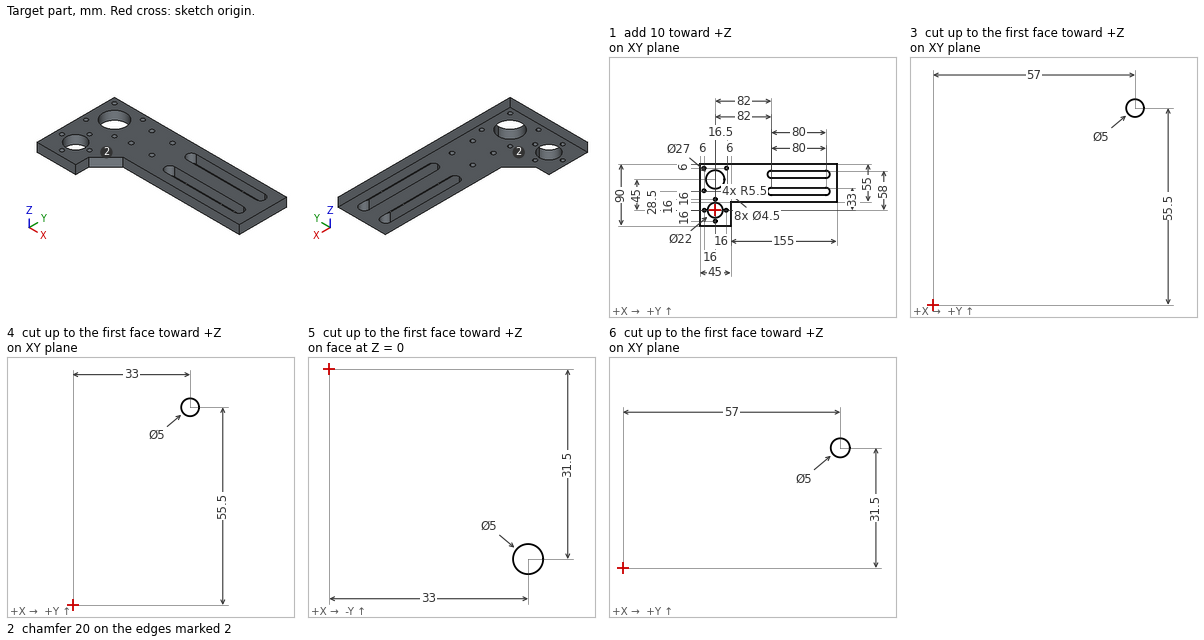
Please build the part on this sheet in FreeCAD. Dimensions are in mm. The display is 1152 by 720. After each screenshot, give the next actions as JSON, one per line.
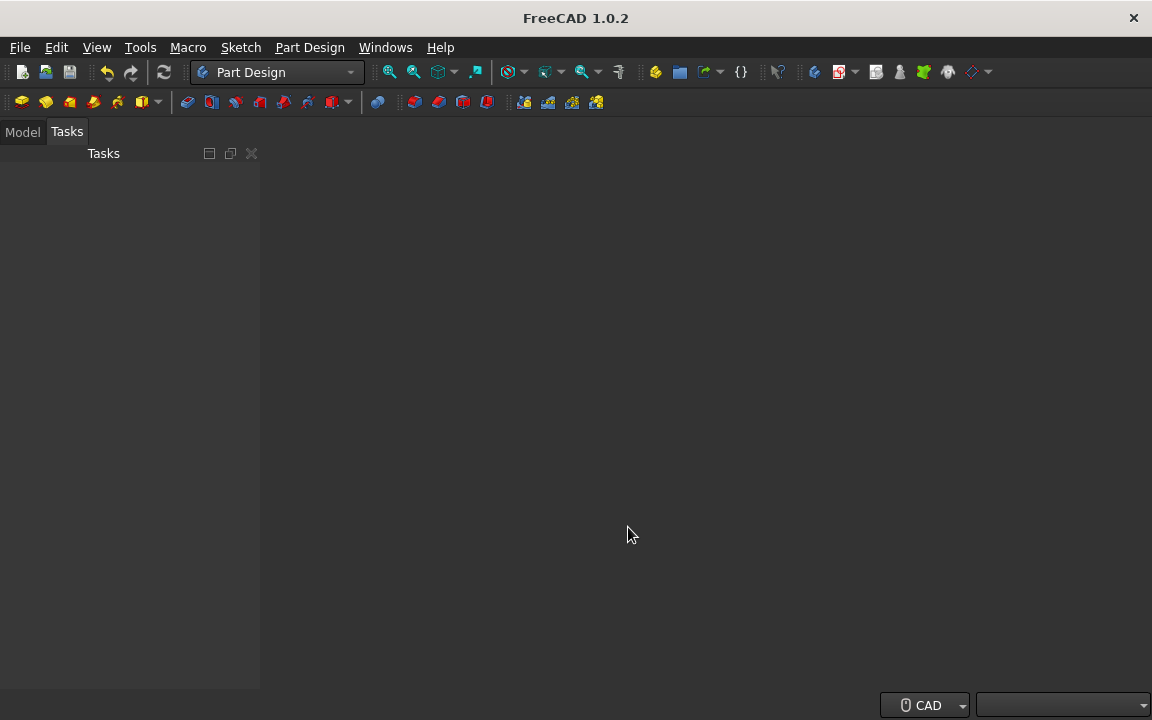
{"action": "key", "text": "ctrl+n"}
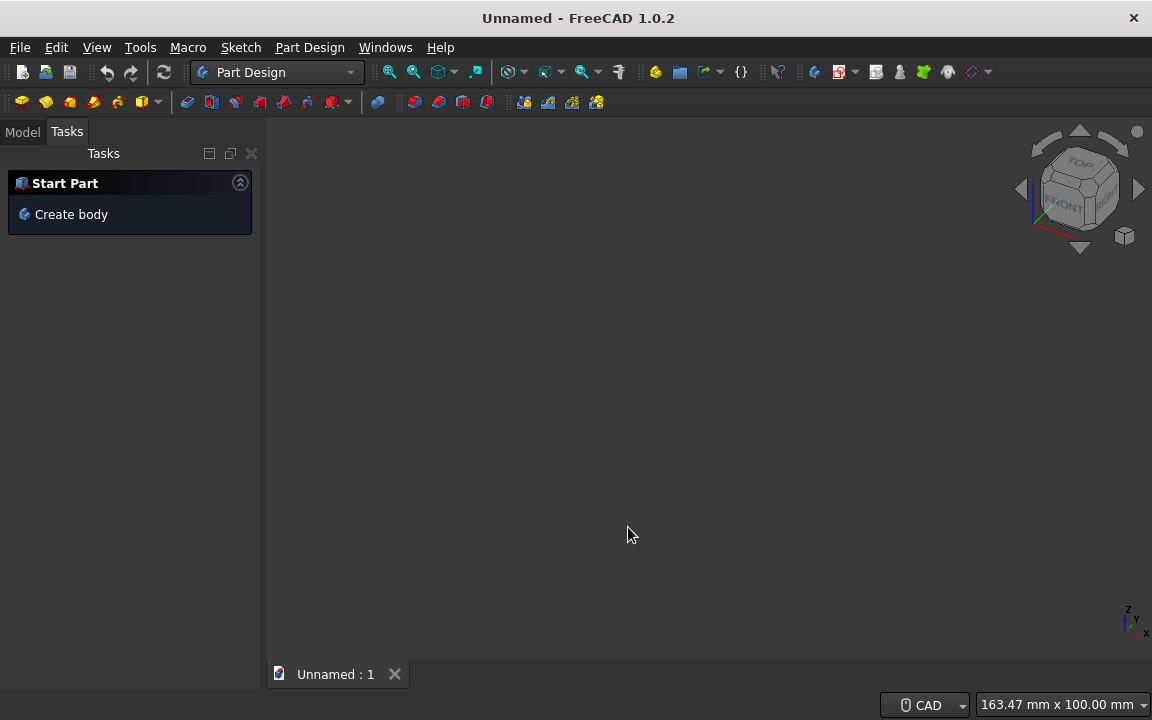
{"action": "left_click", "coordinate": [840, 72]}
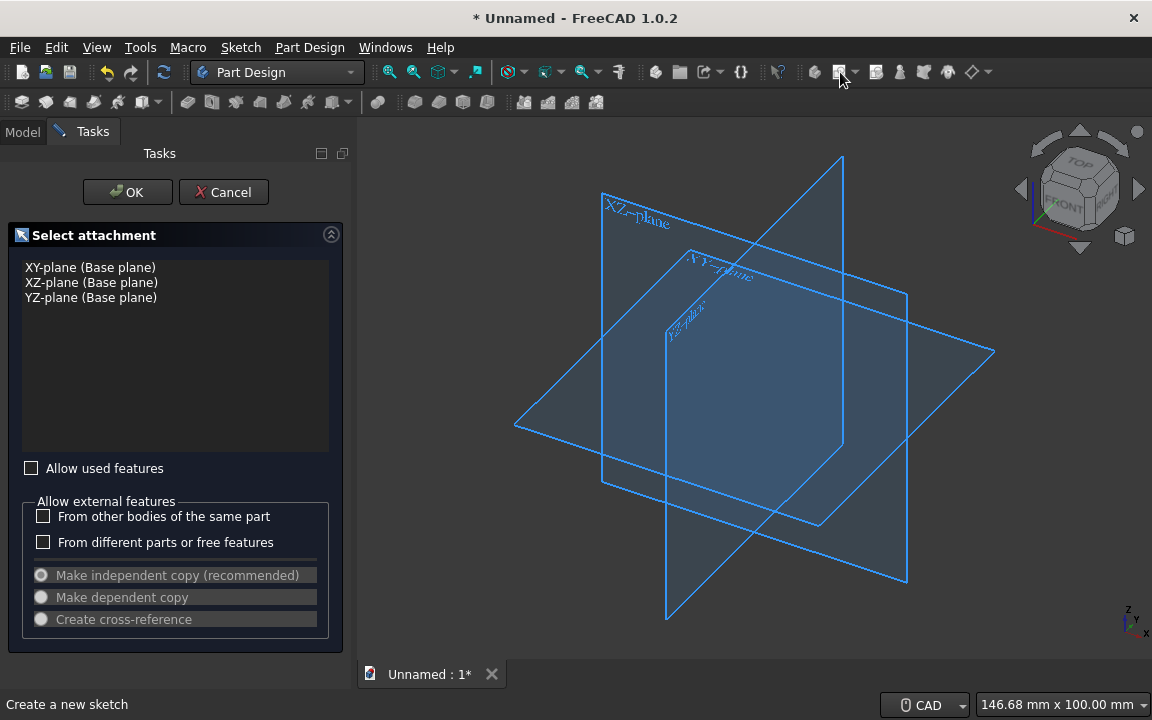
{"action": "left_click", "coordinate": [82, 268]}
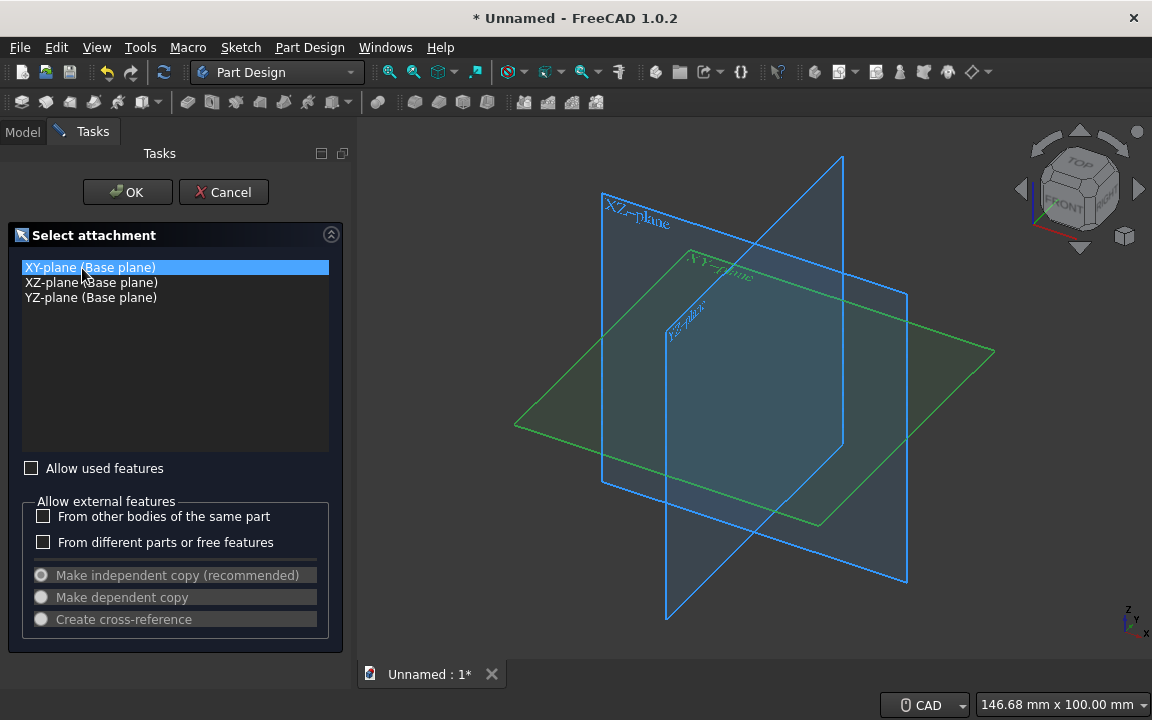
{"action": "left_click", "coordinate": [128, 192]}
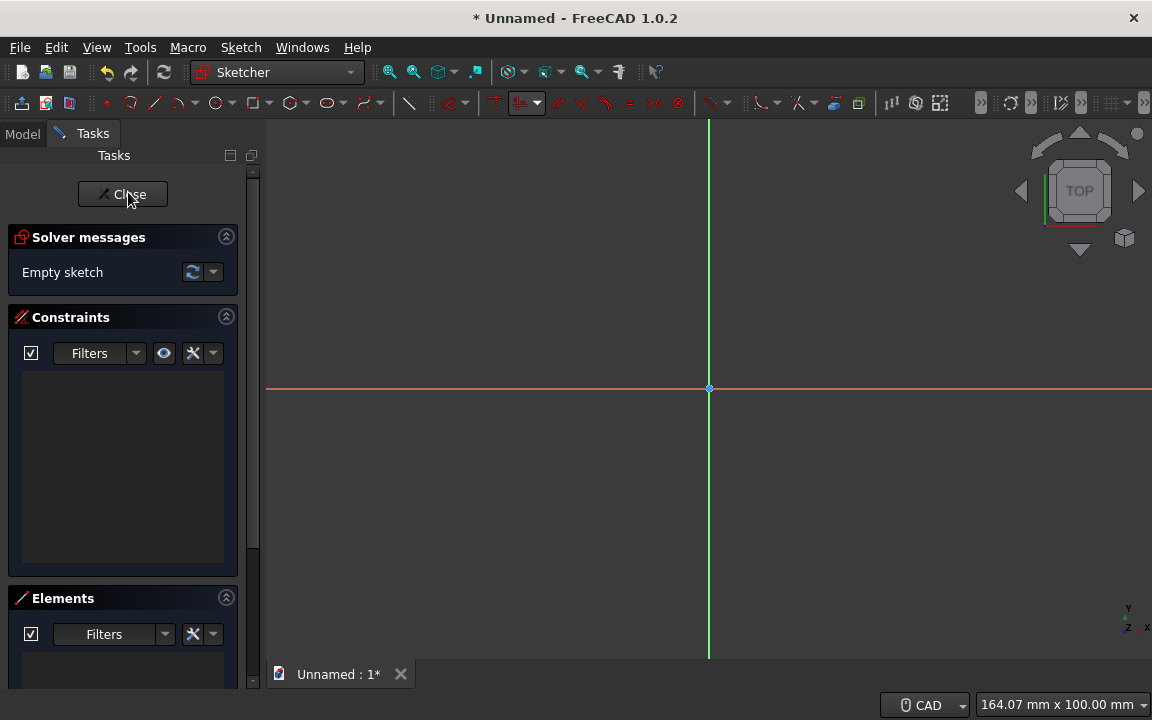
{"action": "scroll", "coordinate": [294, 488], "scroll_direction": "down", "scroll_amount": 4}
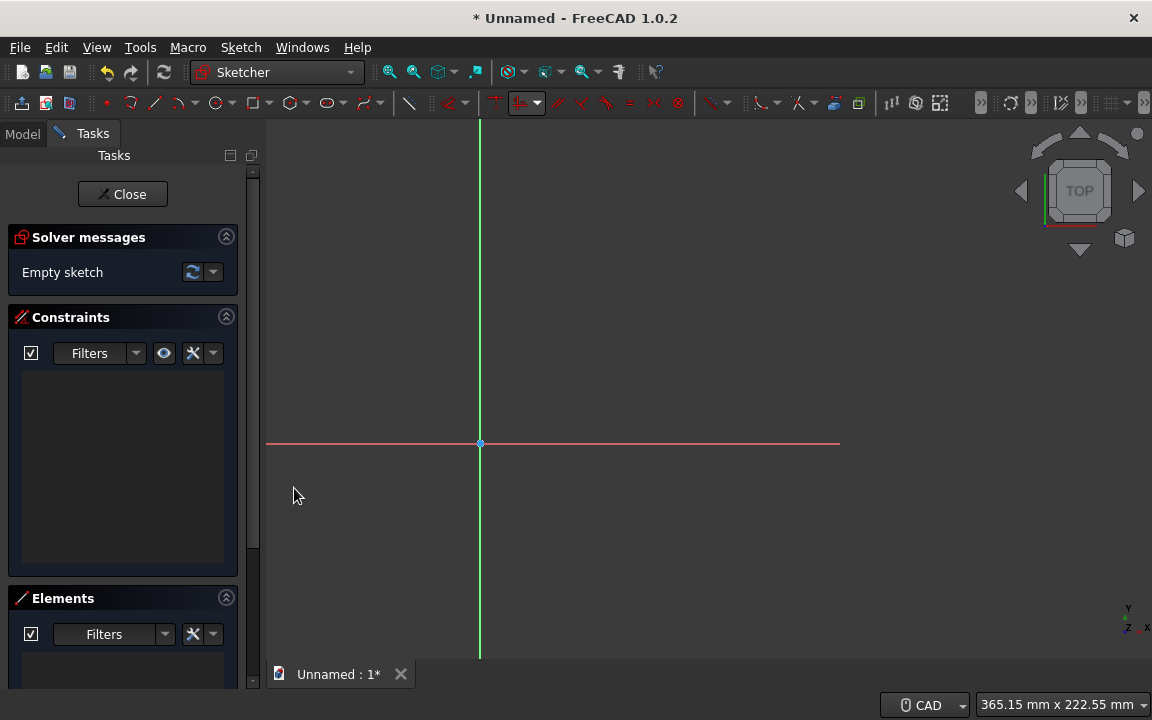
{"action": "key", "text": "g m"}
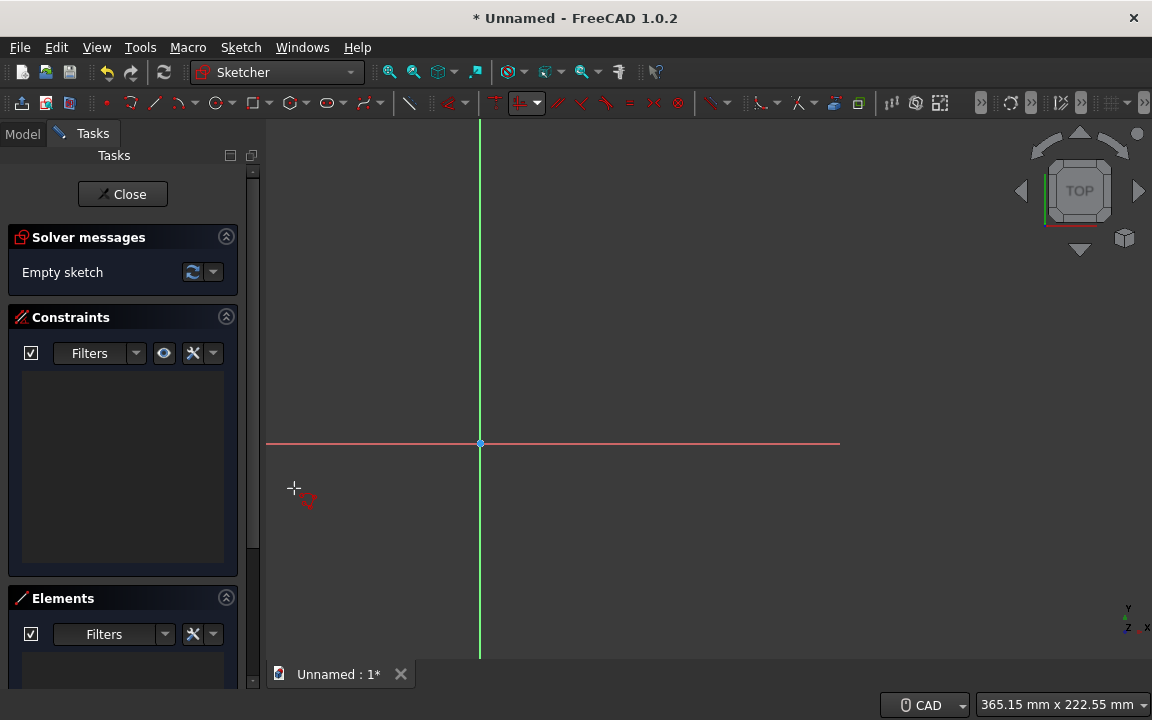
{"action": "left_click", "coordinate": [535, 414]}
{"action": "left_click", "coordinate": [911, 414]}
{"action": "left_click", "coordinate": [911, 280]}
{"action": "left_click", "coordinate": [426, 280]}
{"action": "left_click", "coordinate": [426, 498]}
{"action": "left_click", "coordinate": [535, 498]}
{"action": "left_click", "coordinate": [535, 415]}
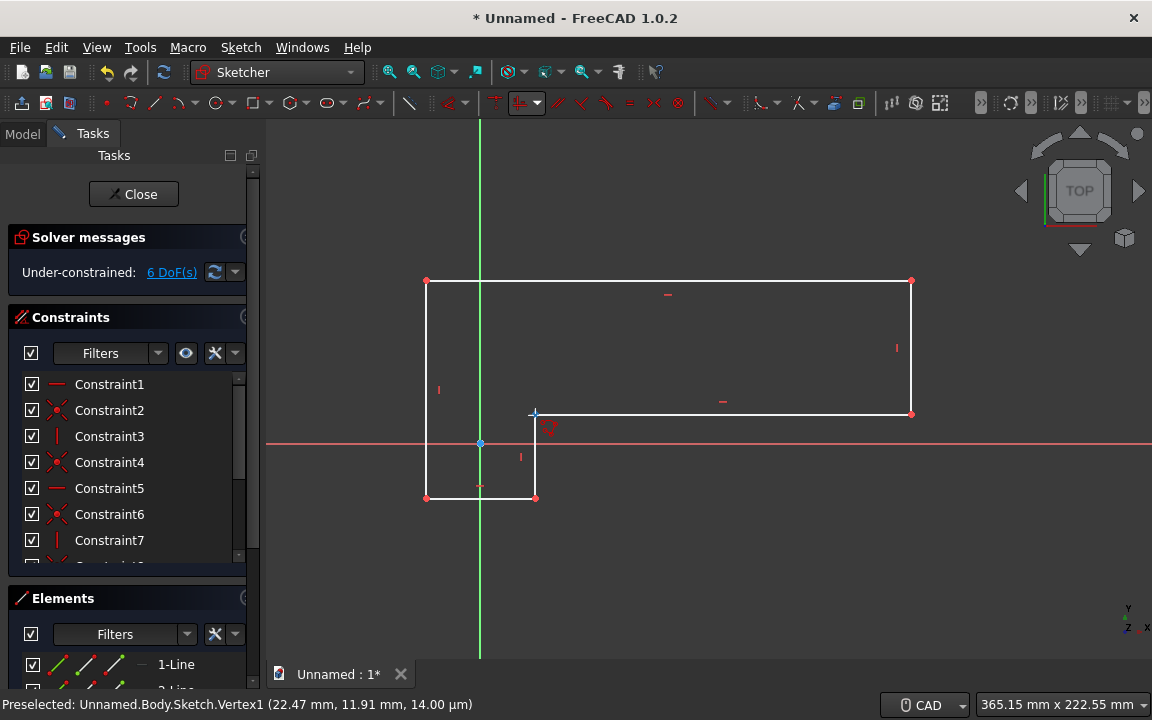
{"action": "key", "text": "g s"}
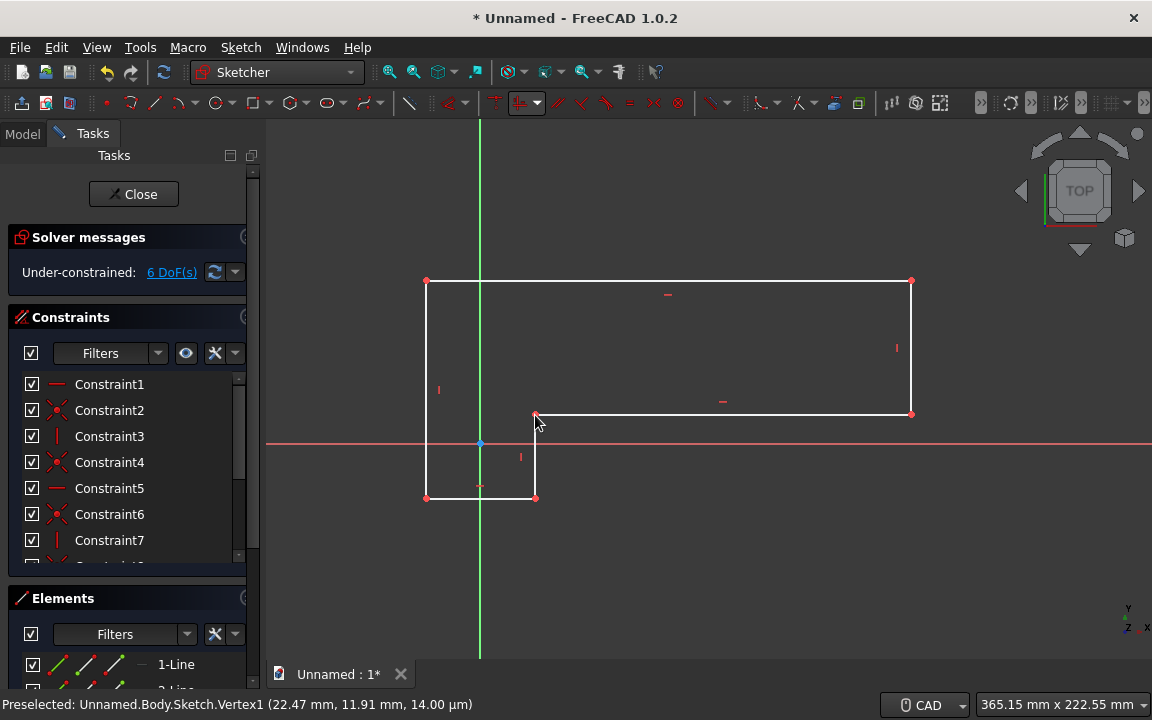
{"action": "scroll", "coordinate": [679, 377], "scroll_direction": "up", "scroll_amount": 3}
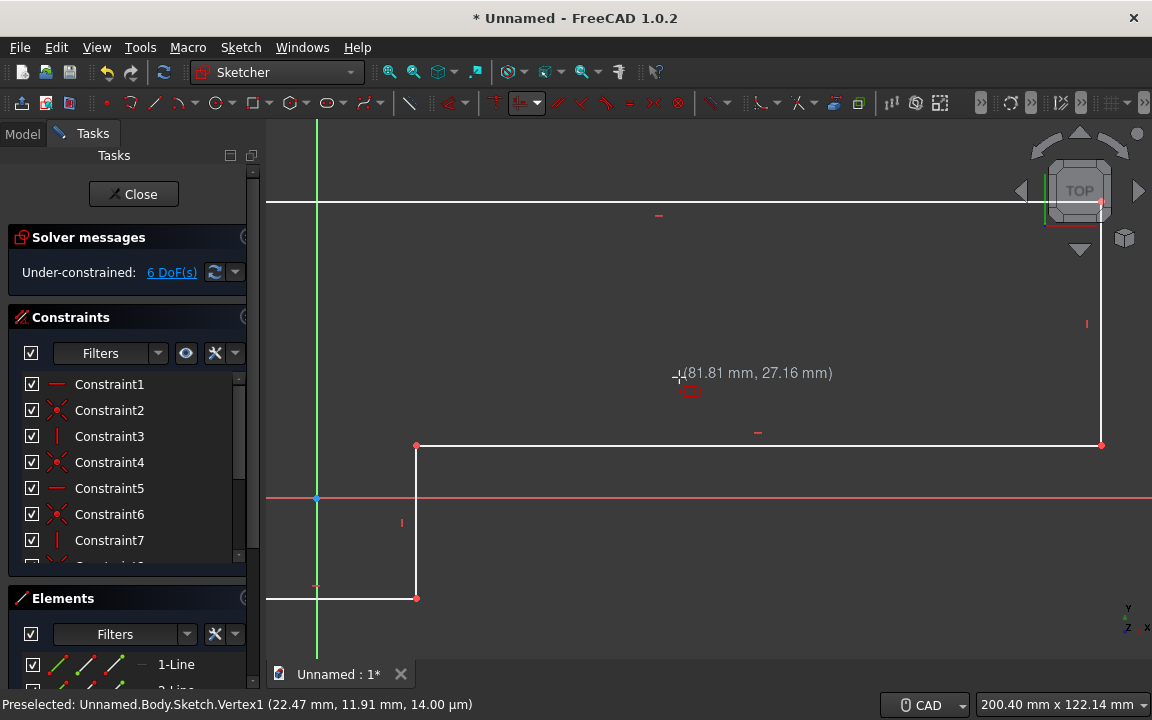
{"action": "left_click", "coordinate": [679, 377]}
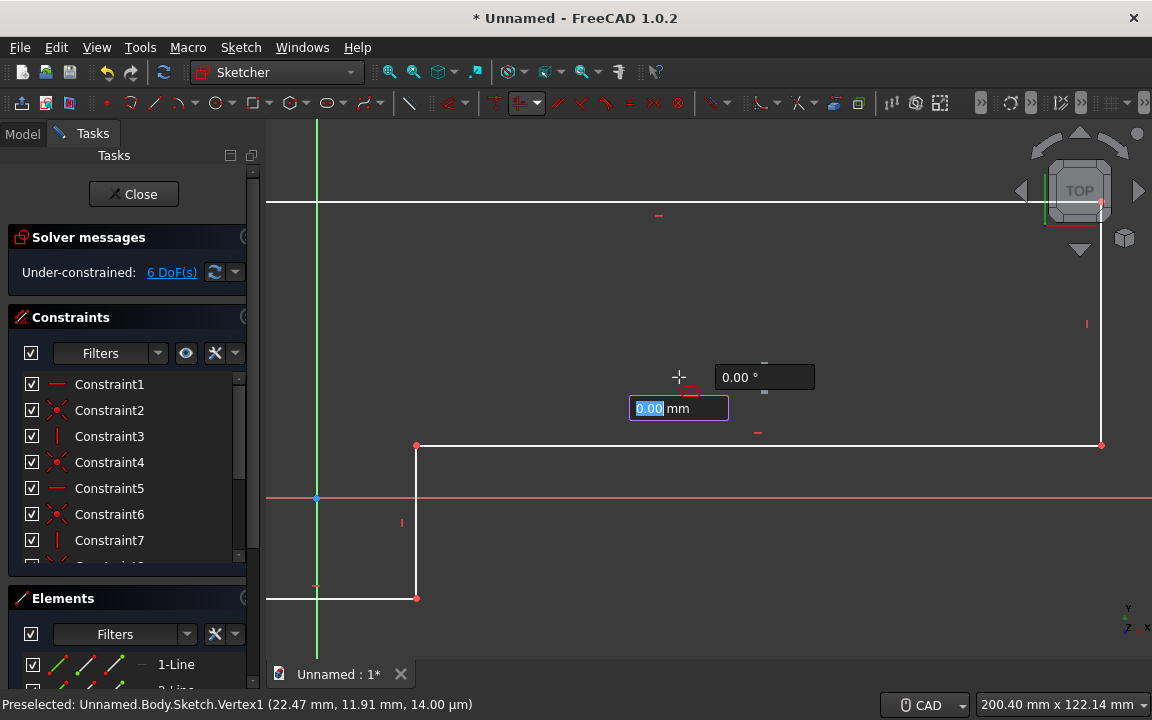
{"action": "scroll", "coordinate": [617, 377], "scroll_direction": "down", "scroll_amount": 3}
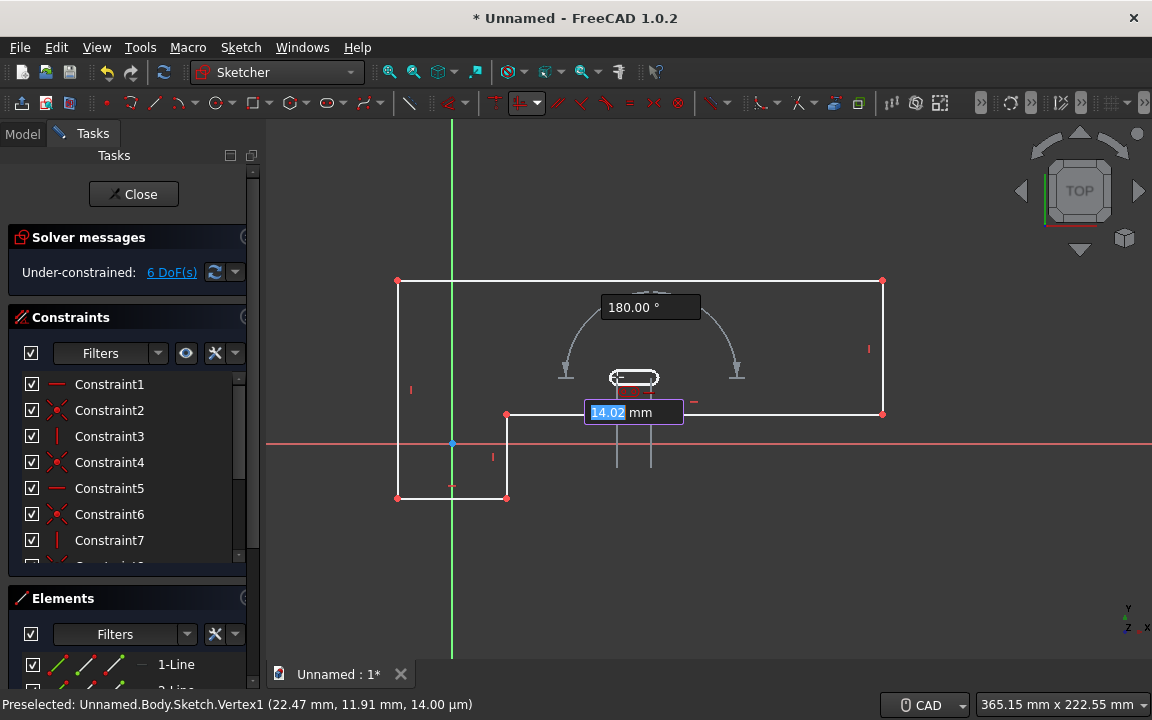
{"action": "left_click", "coordinate": [846, 377]}